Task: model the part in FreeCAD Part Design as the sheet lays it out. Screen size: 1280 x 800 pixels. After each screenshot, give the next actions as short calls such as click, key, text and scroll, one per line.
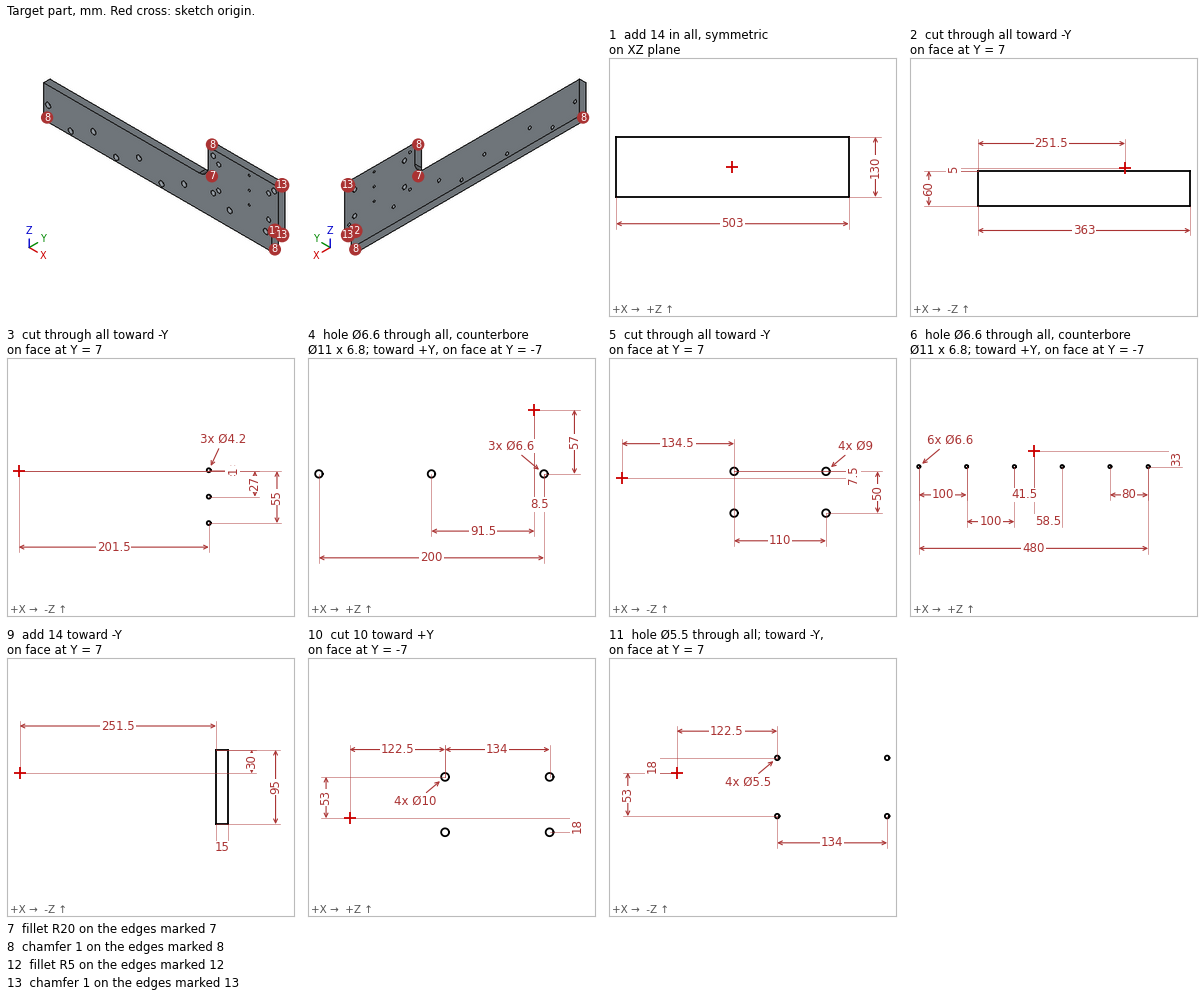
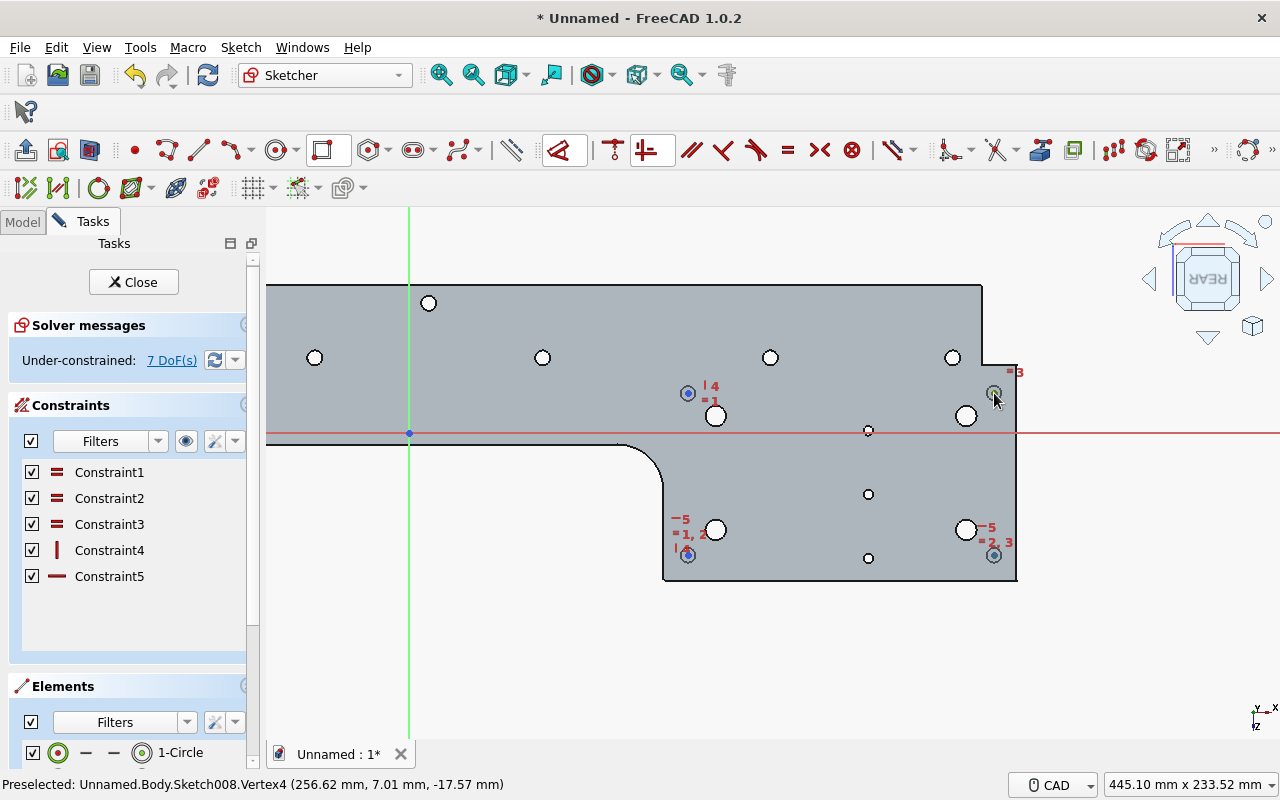
key(v)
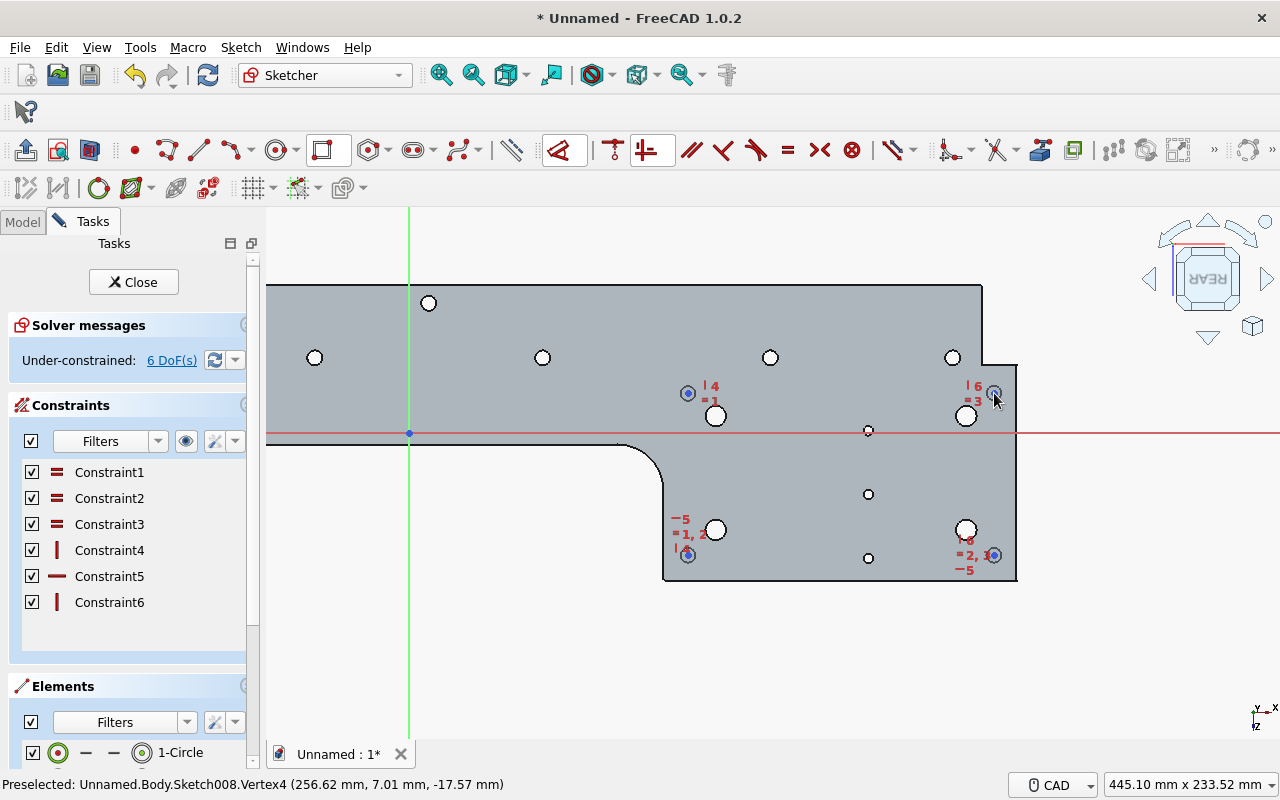
click(688, 393)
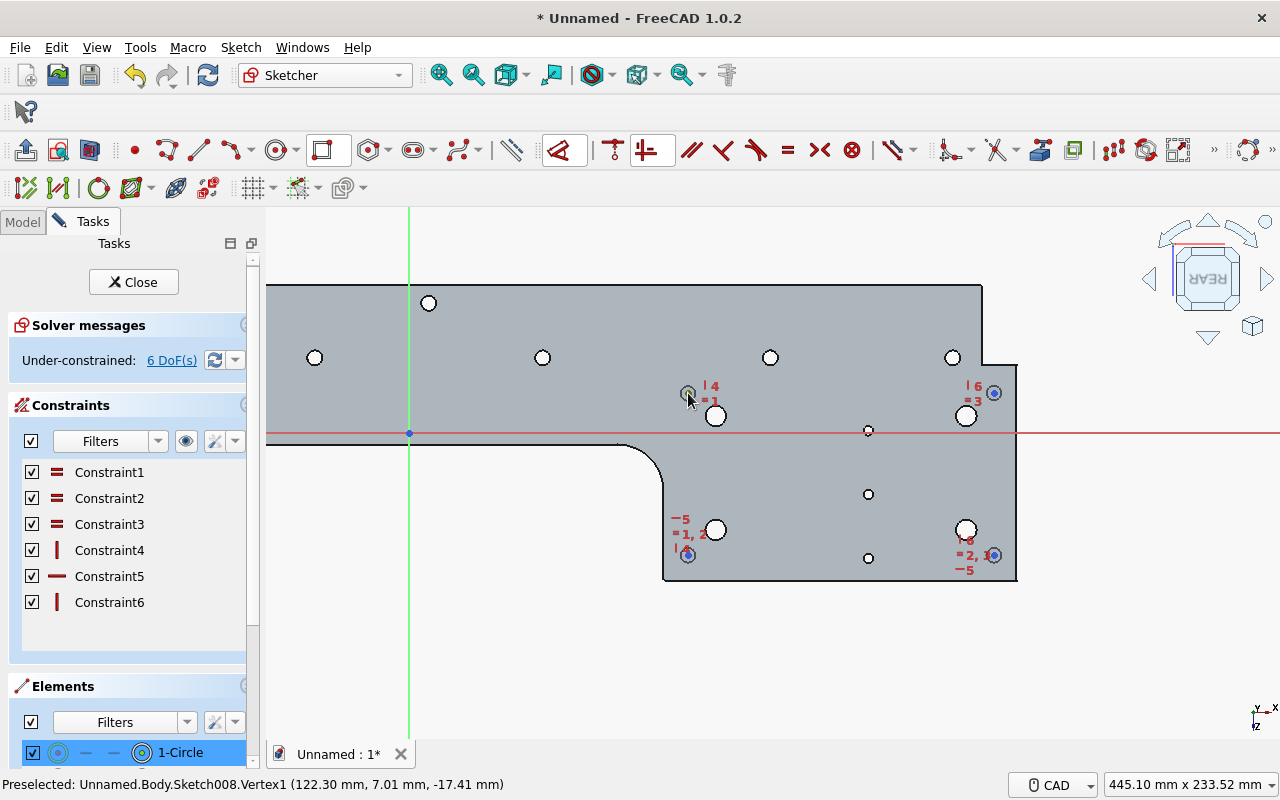
click(994, 393)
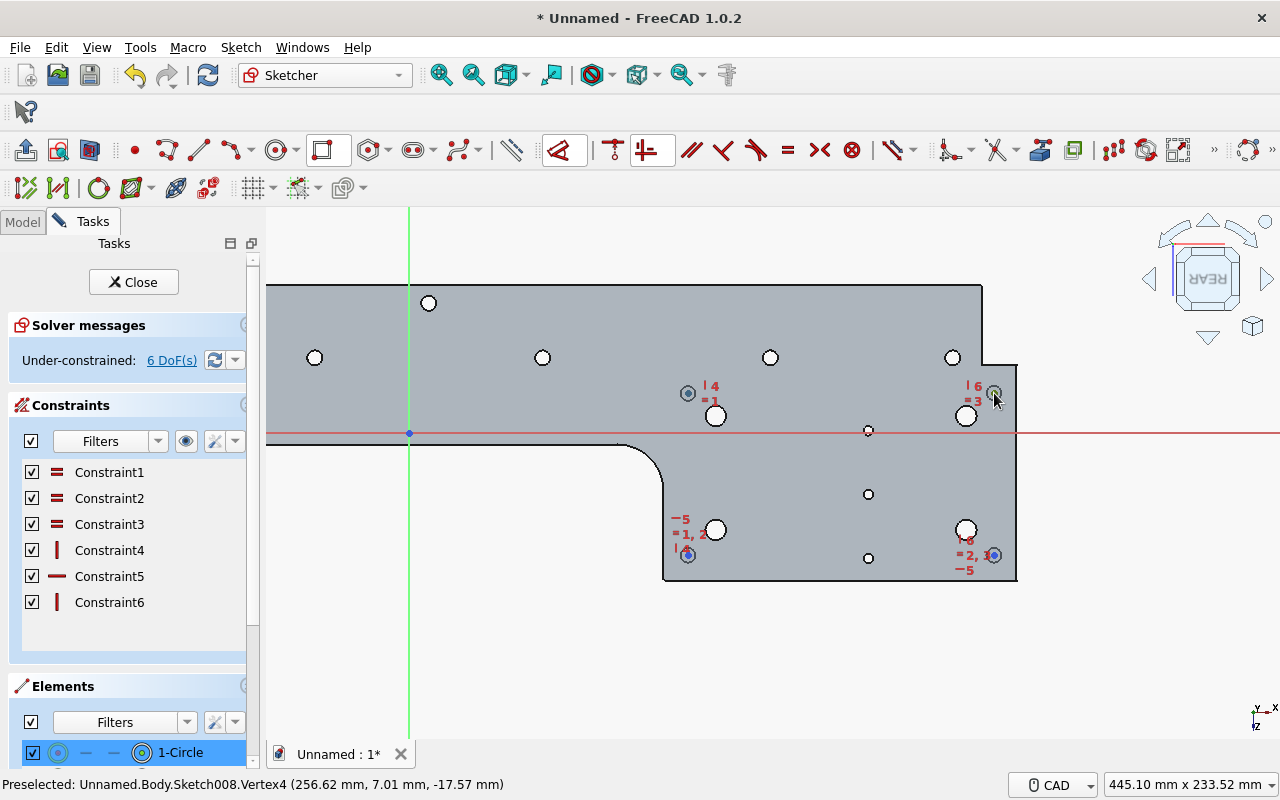
key(h)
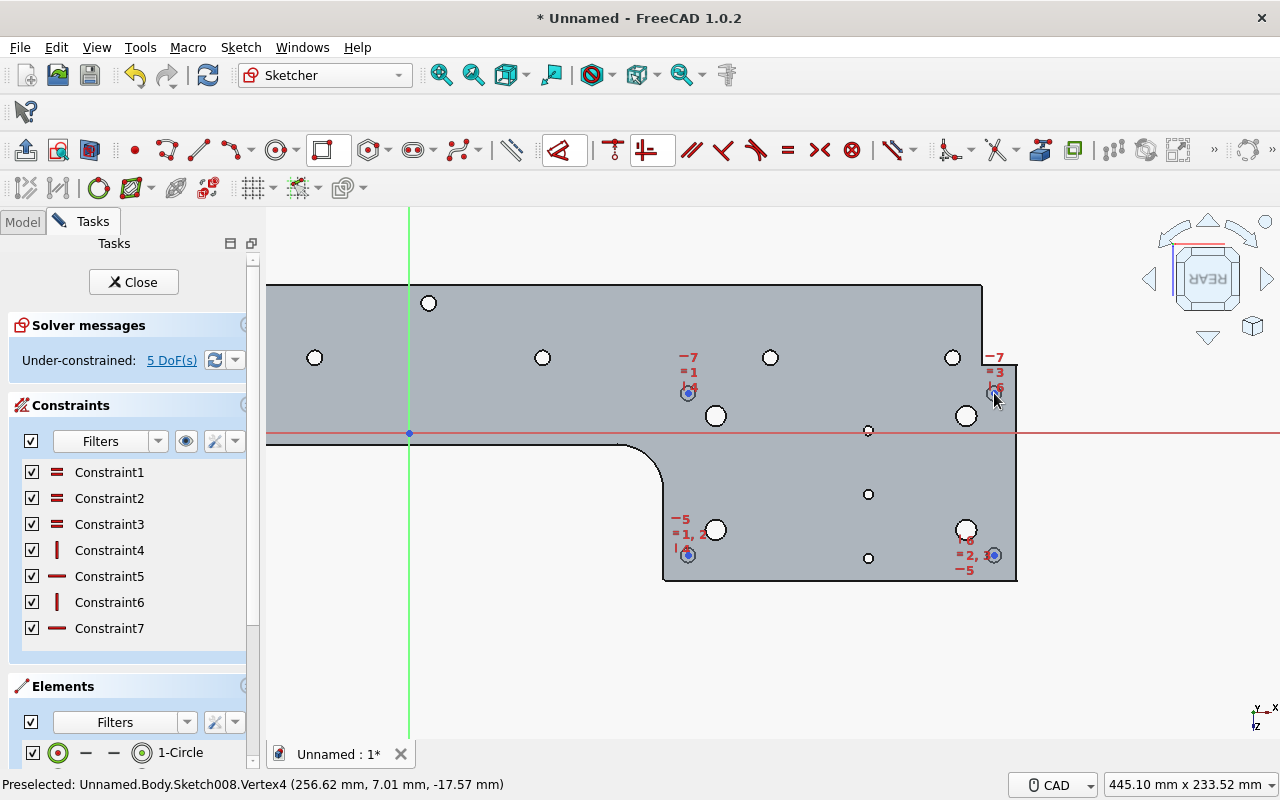
scroll(683, 388, up, 6)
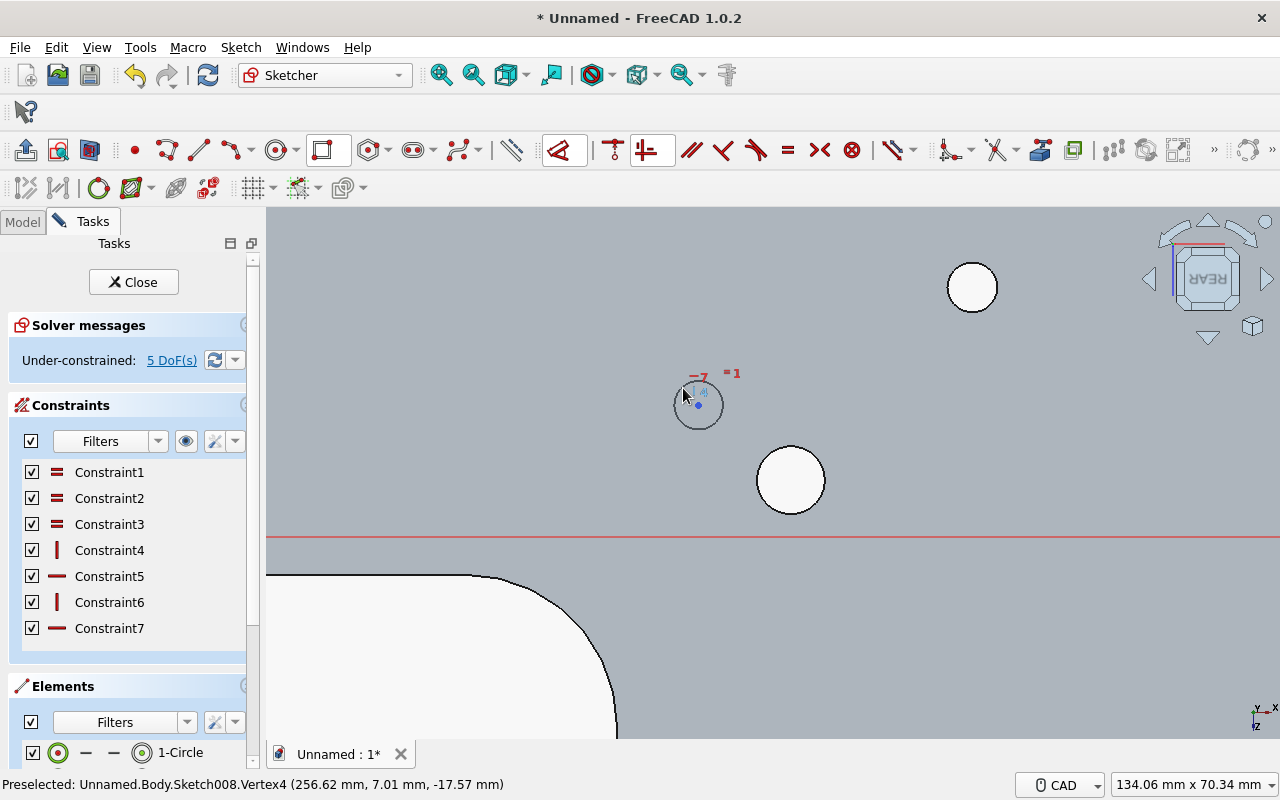
click(681, 388)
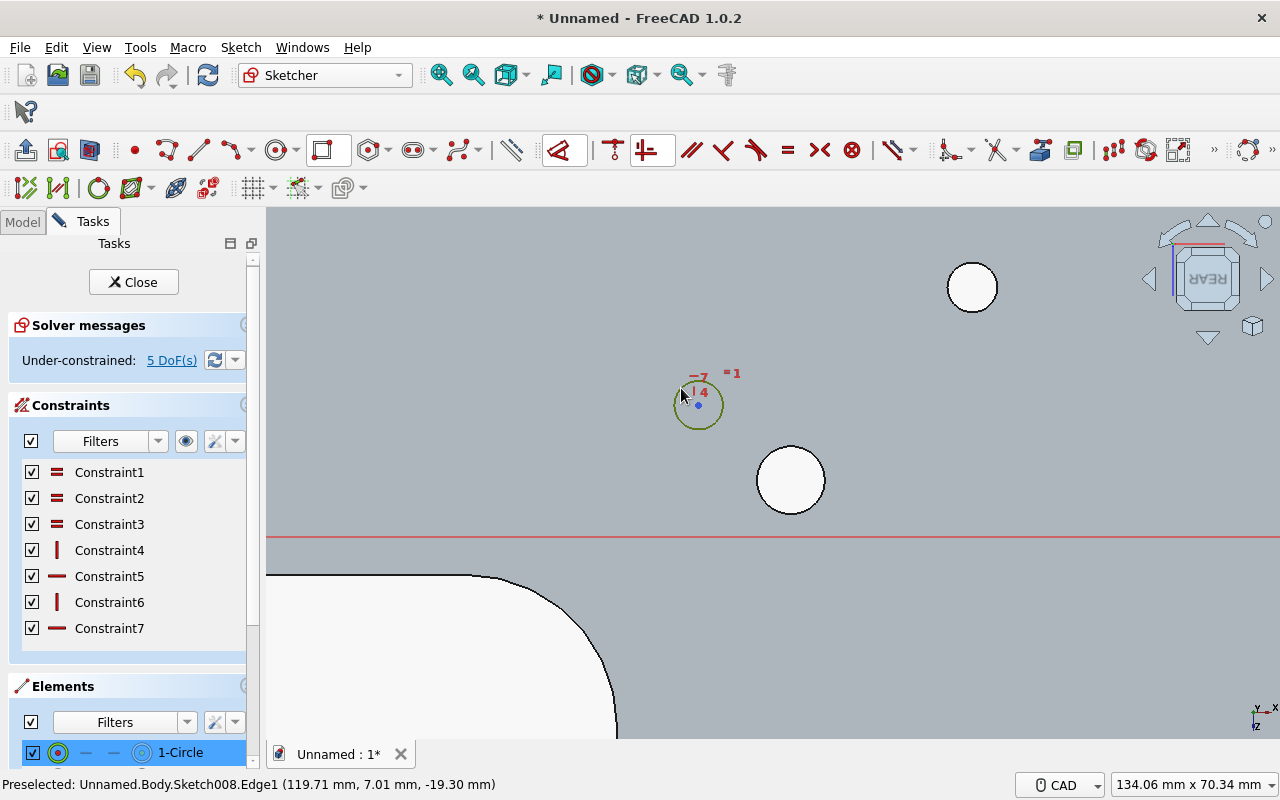
key(k)
key(o)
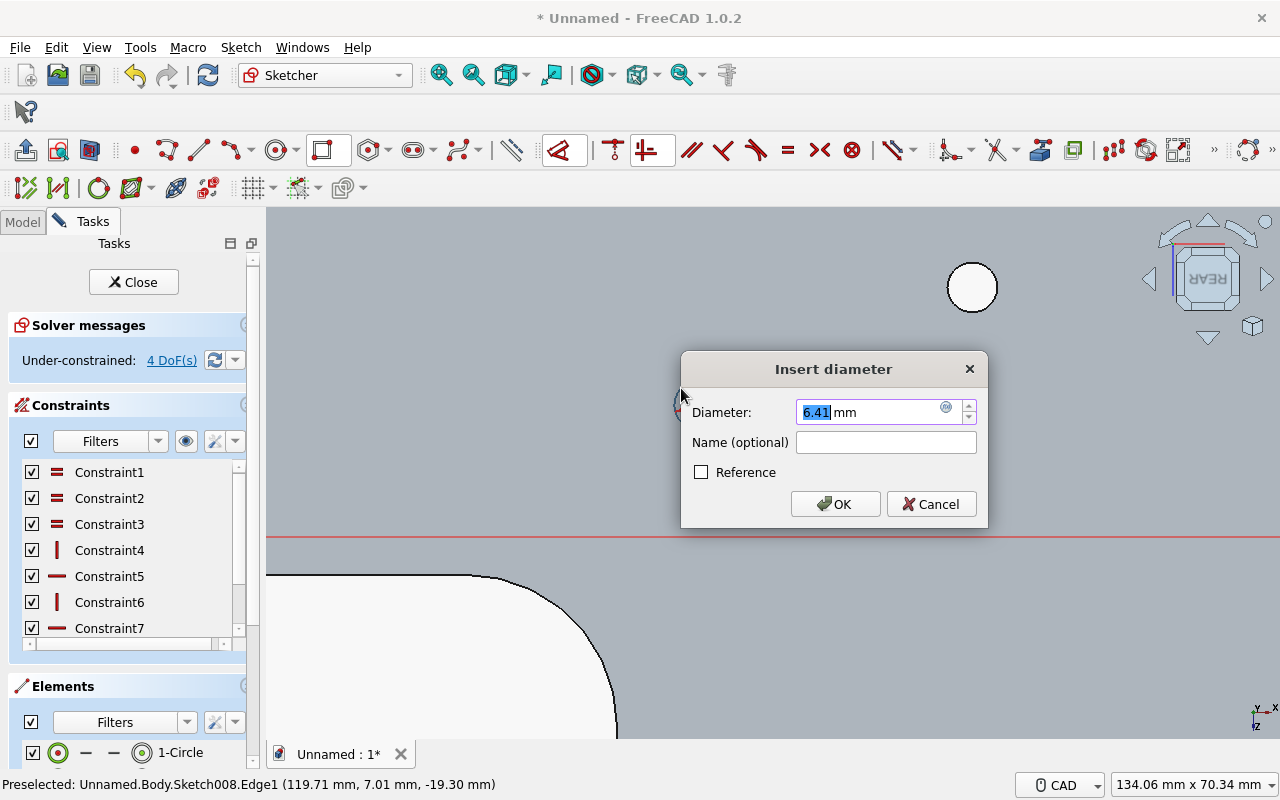
text(5.5)
key(Return)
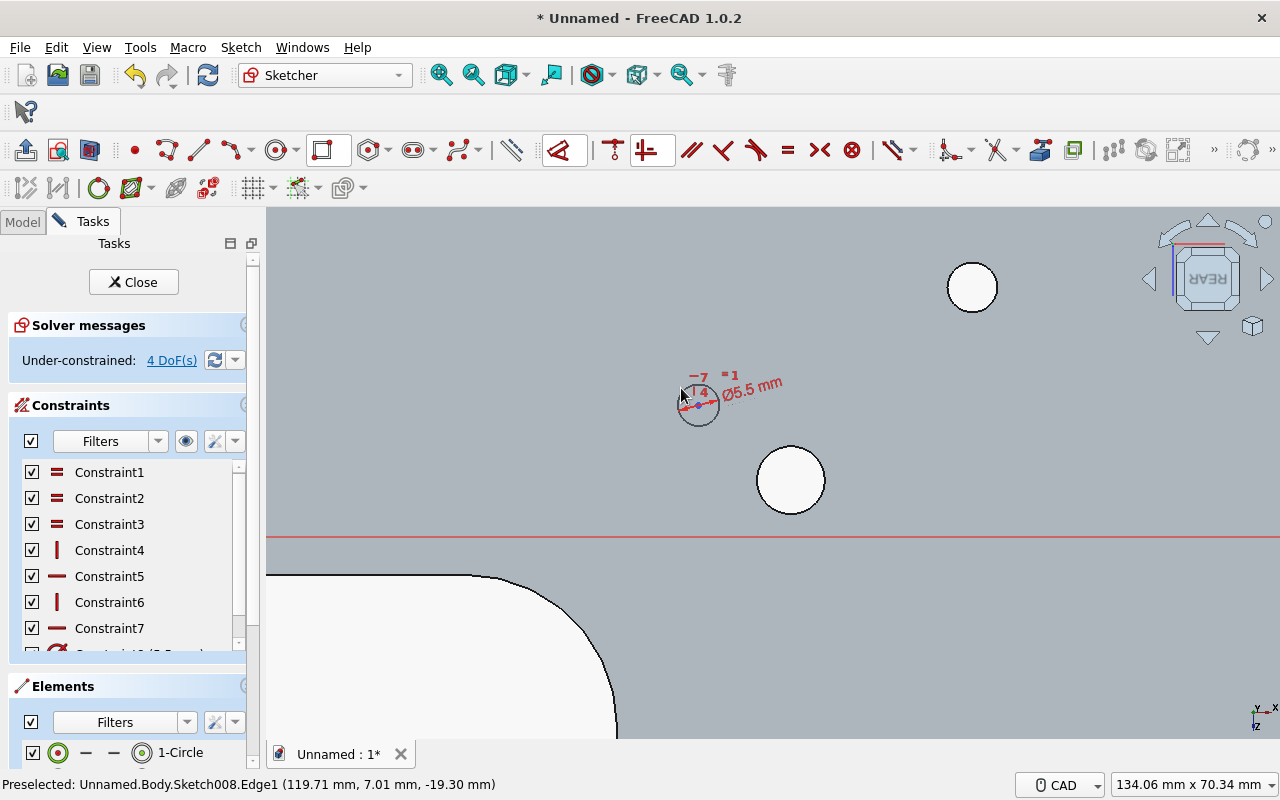
click(699, 405)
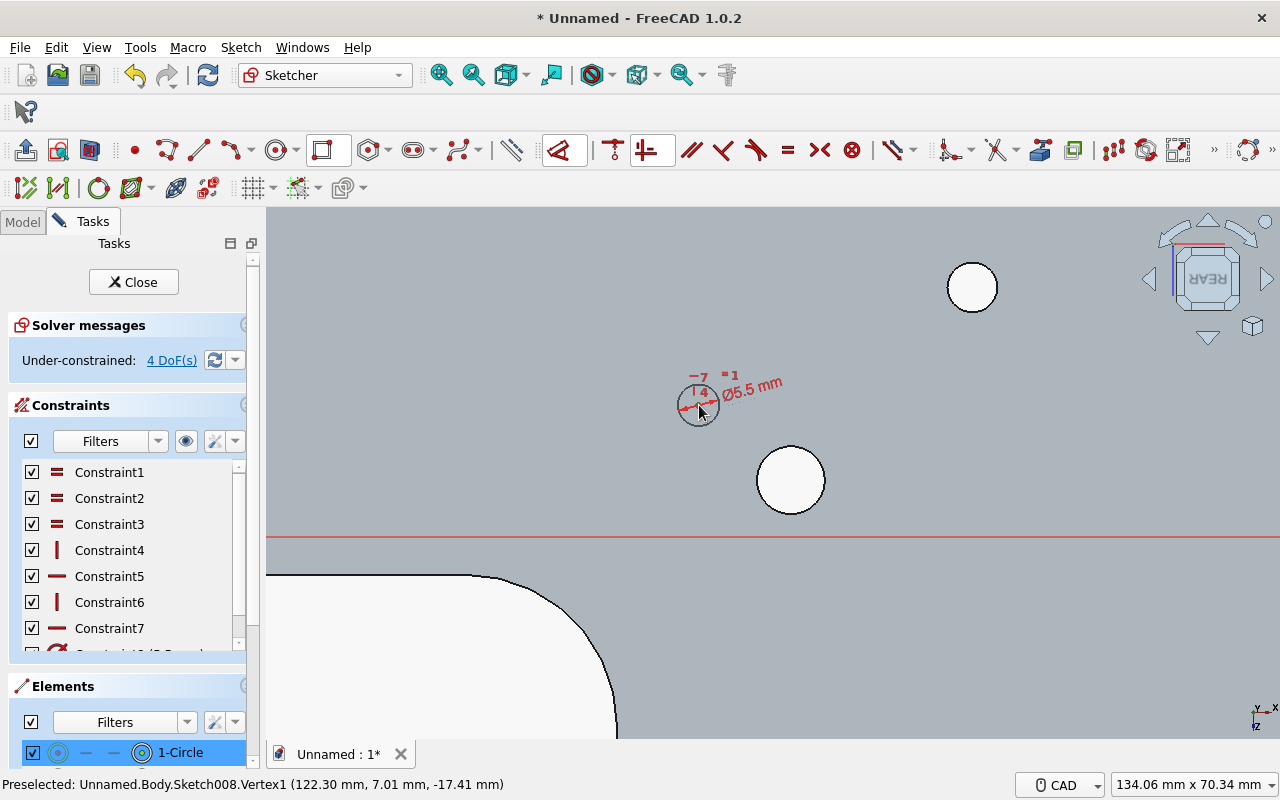
key(i)